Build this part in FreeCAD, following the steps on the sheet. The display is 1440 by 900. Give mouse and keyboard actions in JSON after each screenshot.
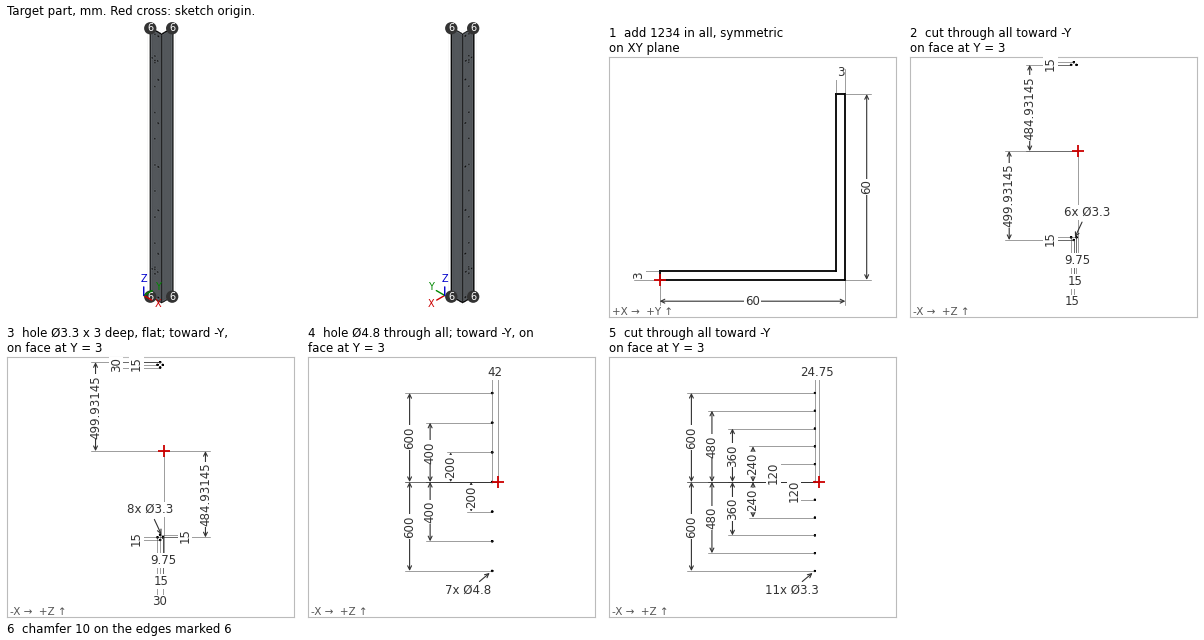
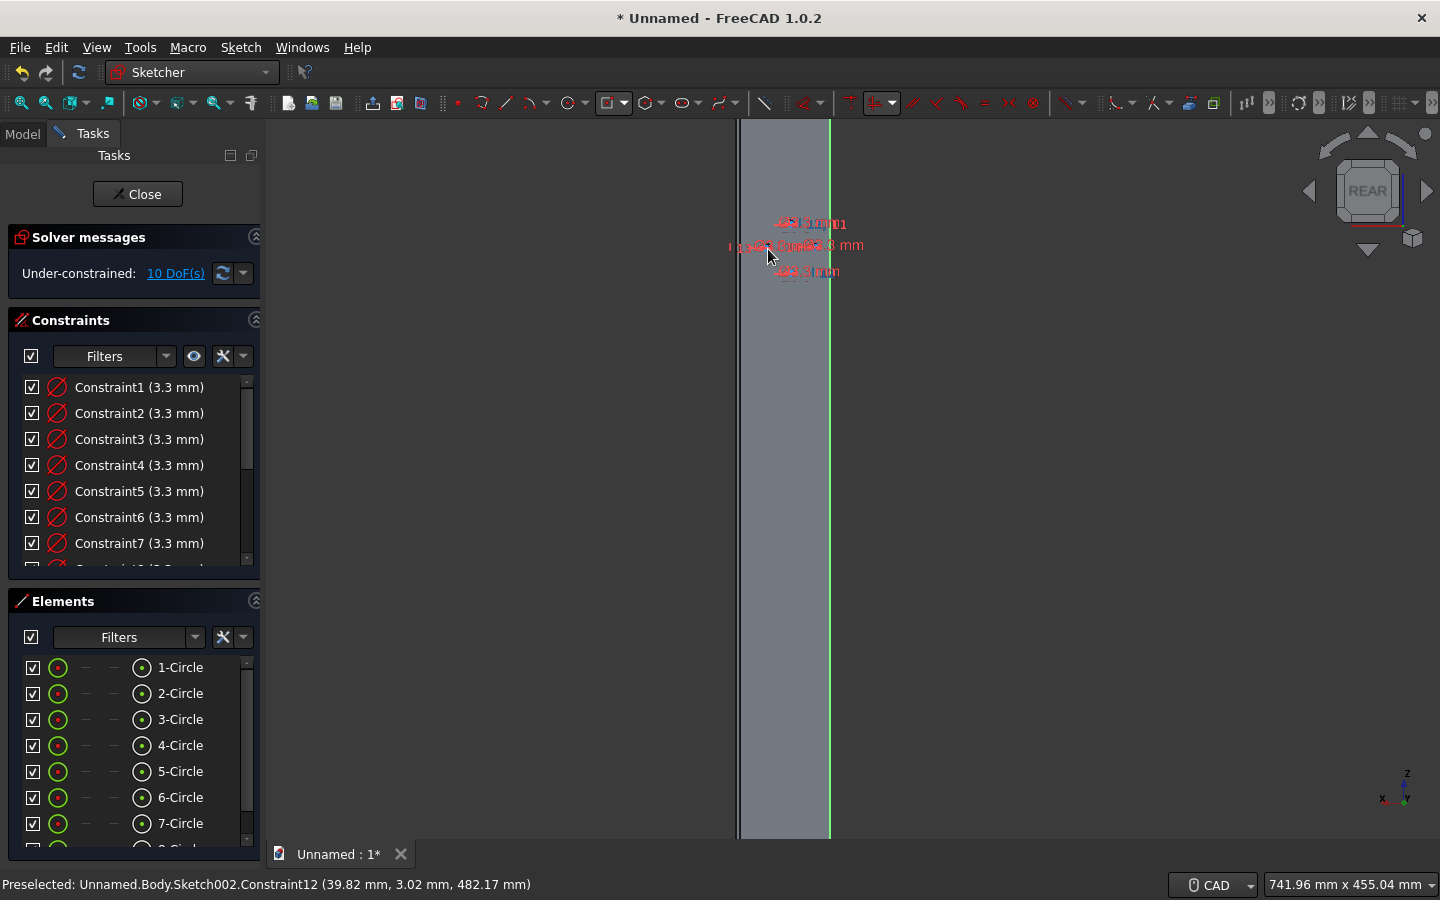
{"action": "left_click", "coordinate": [766, 248]}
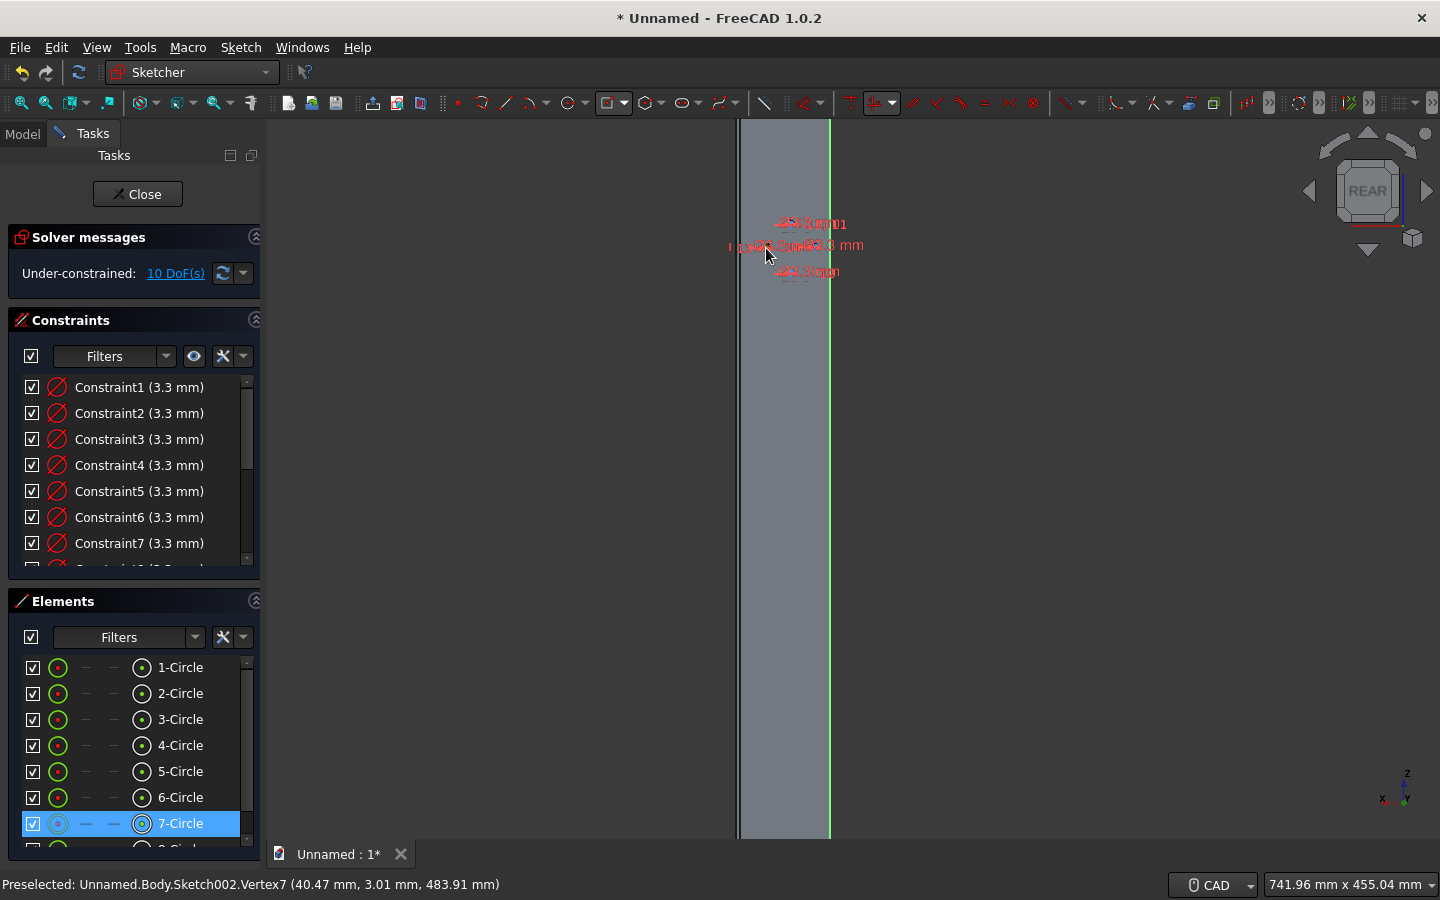
{"action": "left_click", "coordinate": [815, 247]}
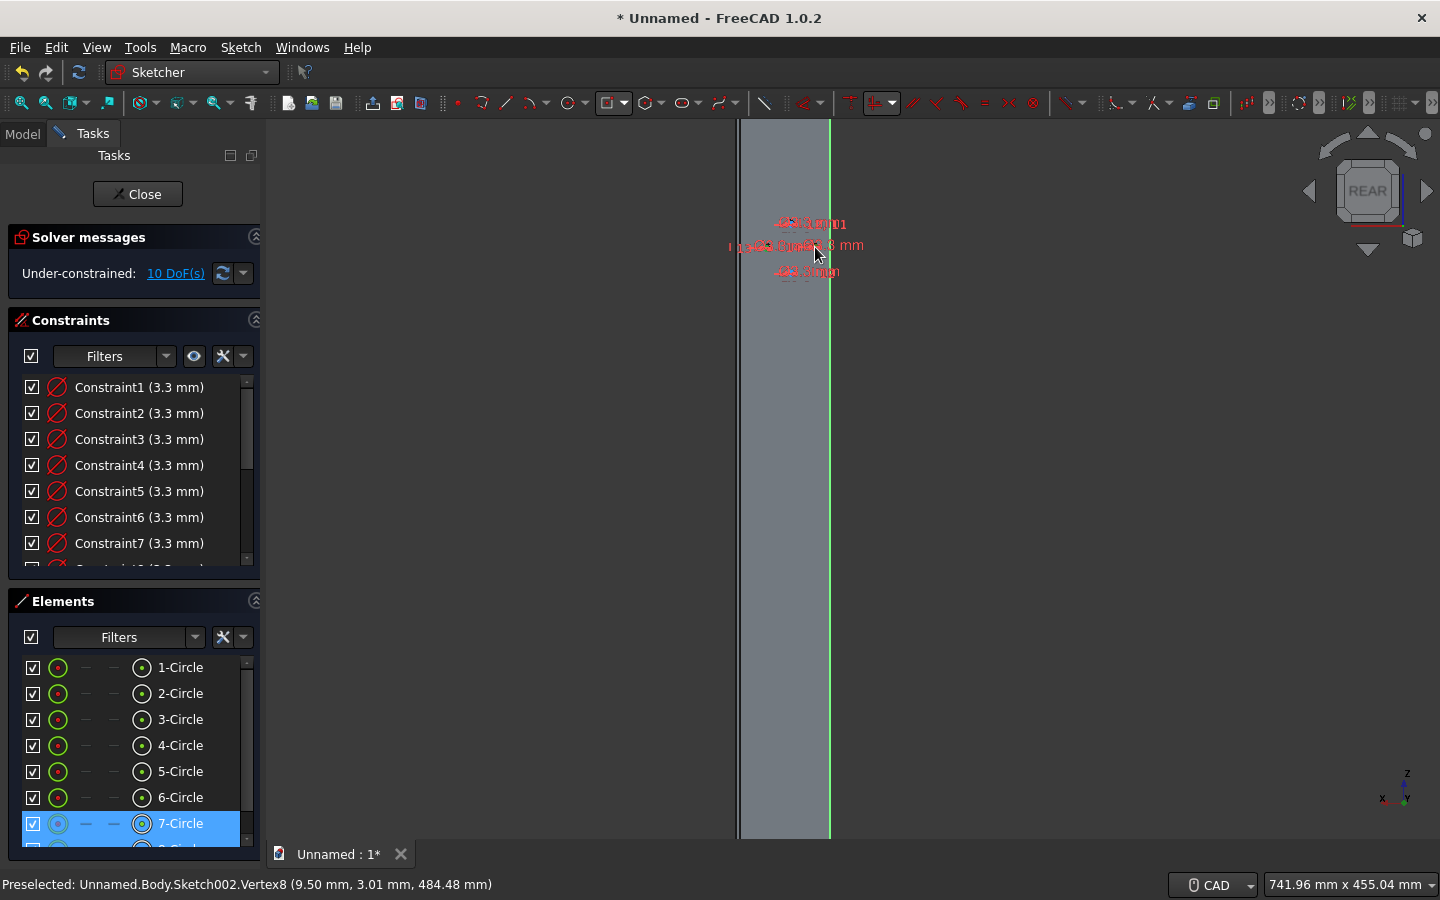
{"action": "left_click", "coordinate": [894, 104]}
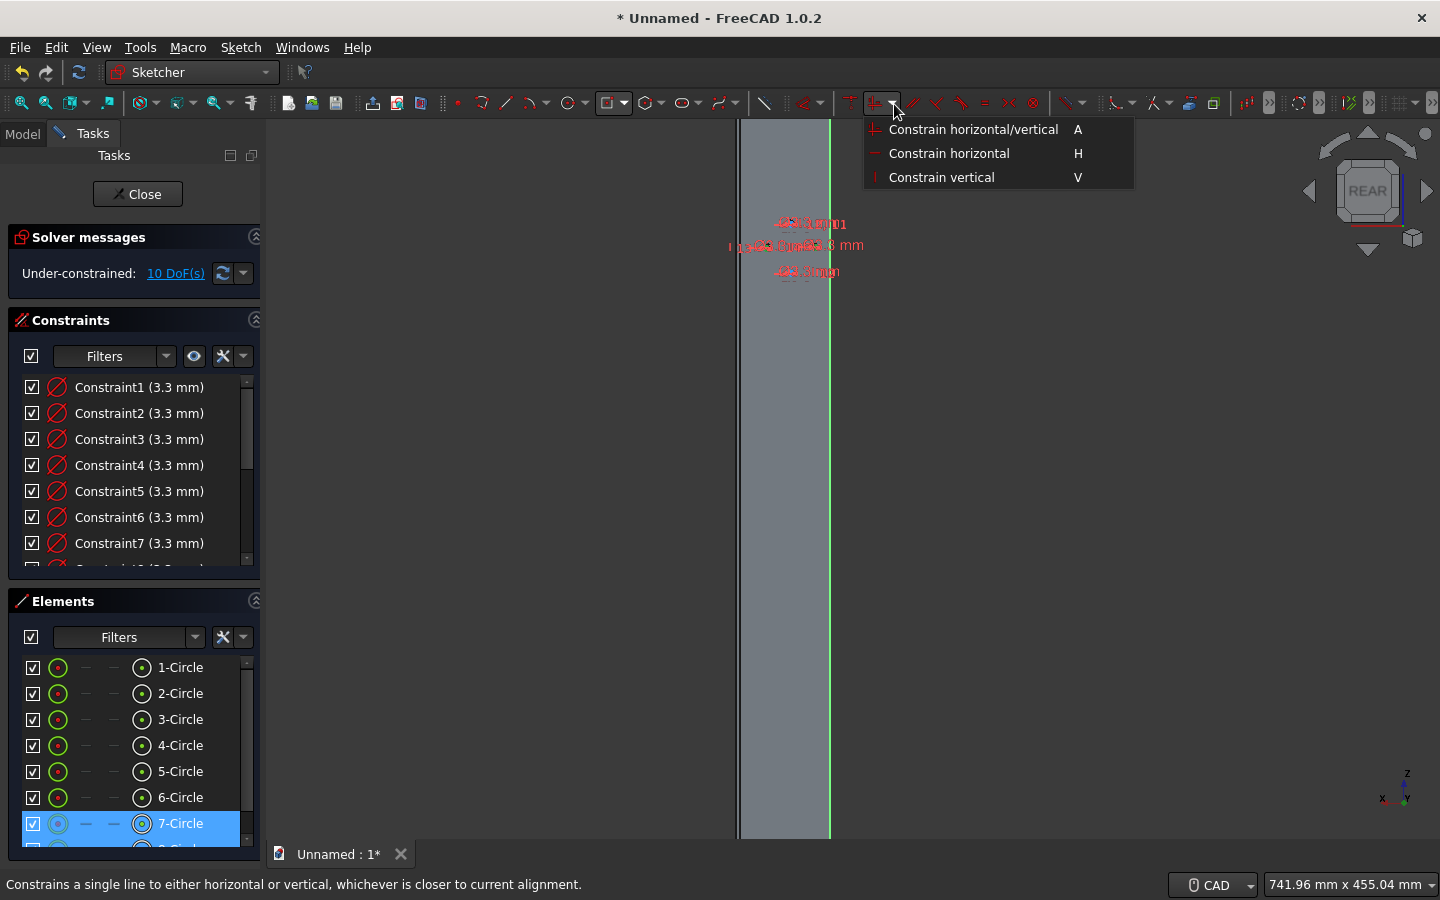
{"action": "left_click", "coordinate": [999, 153]}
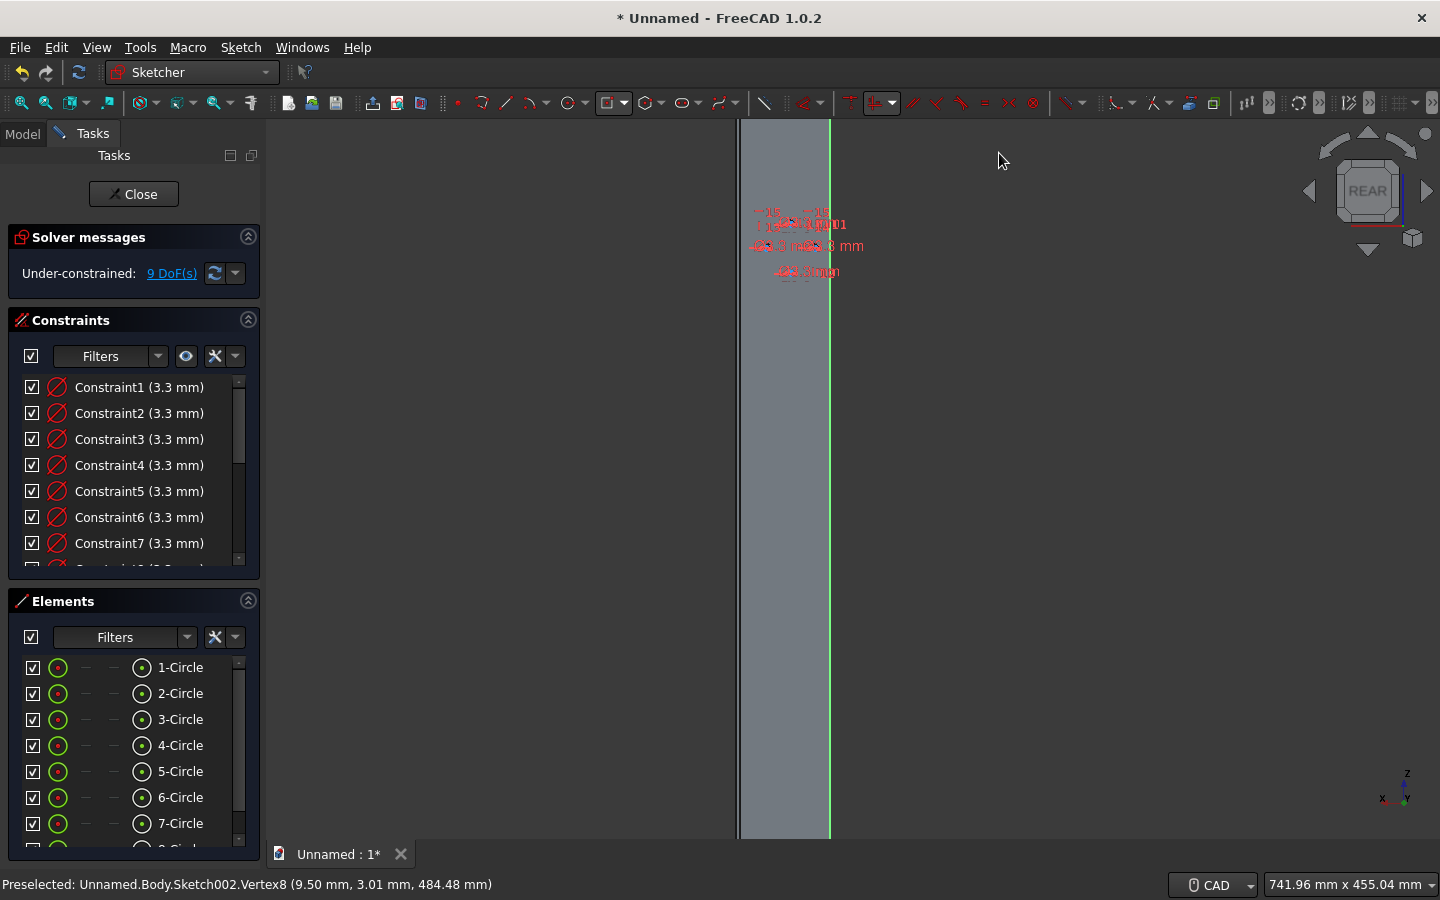
{"action": "left_click", "coordinate": [804, 104]}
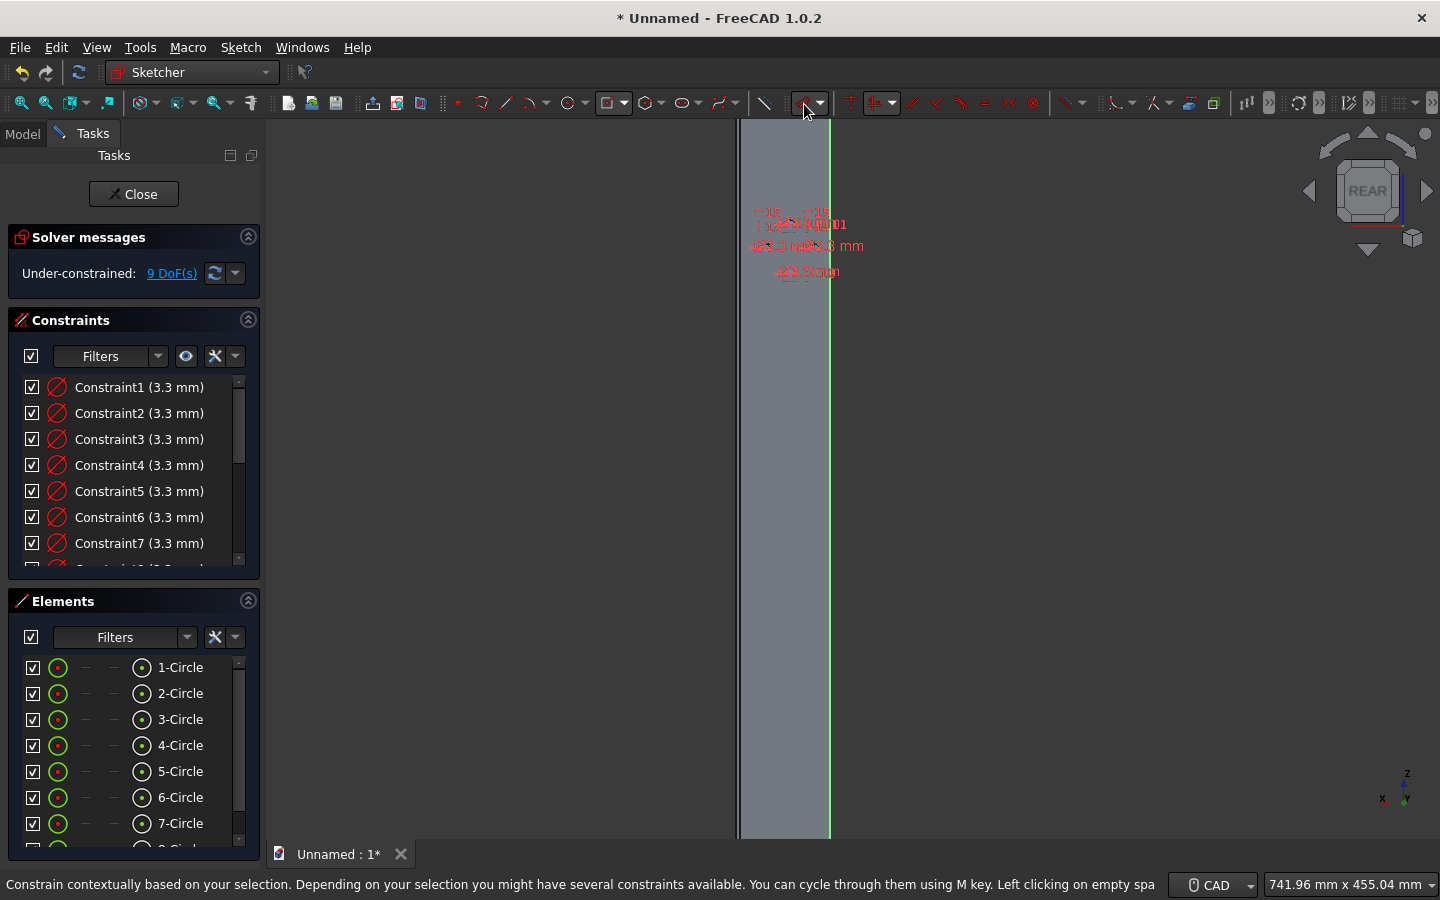
{"action": "scroll", "coordinate": [779, 248], "scroll_direction": "down", "scroll_amount": 6}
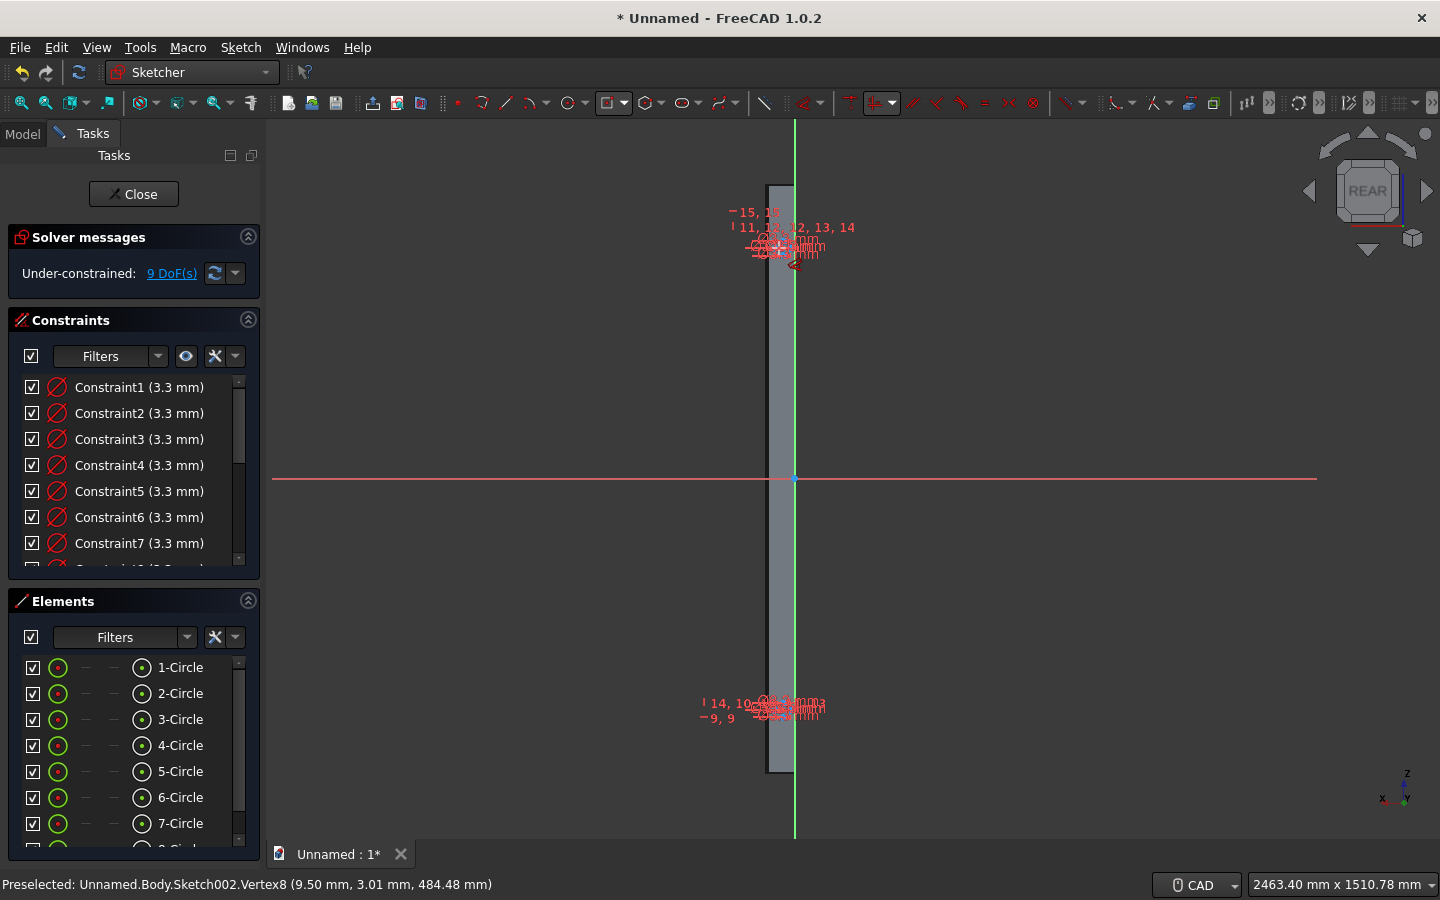
{"action": "scroll", "coordinate": [790, 710], "scroll_direction": "up", "scroll_amount": 6}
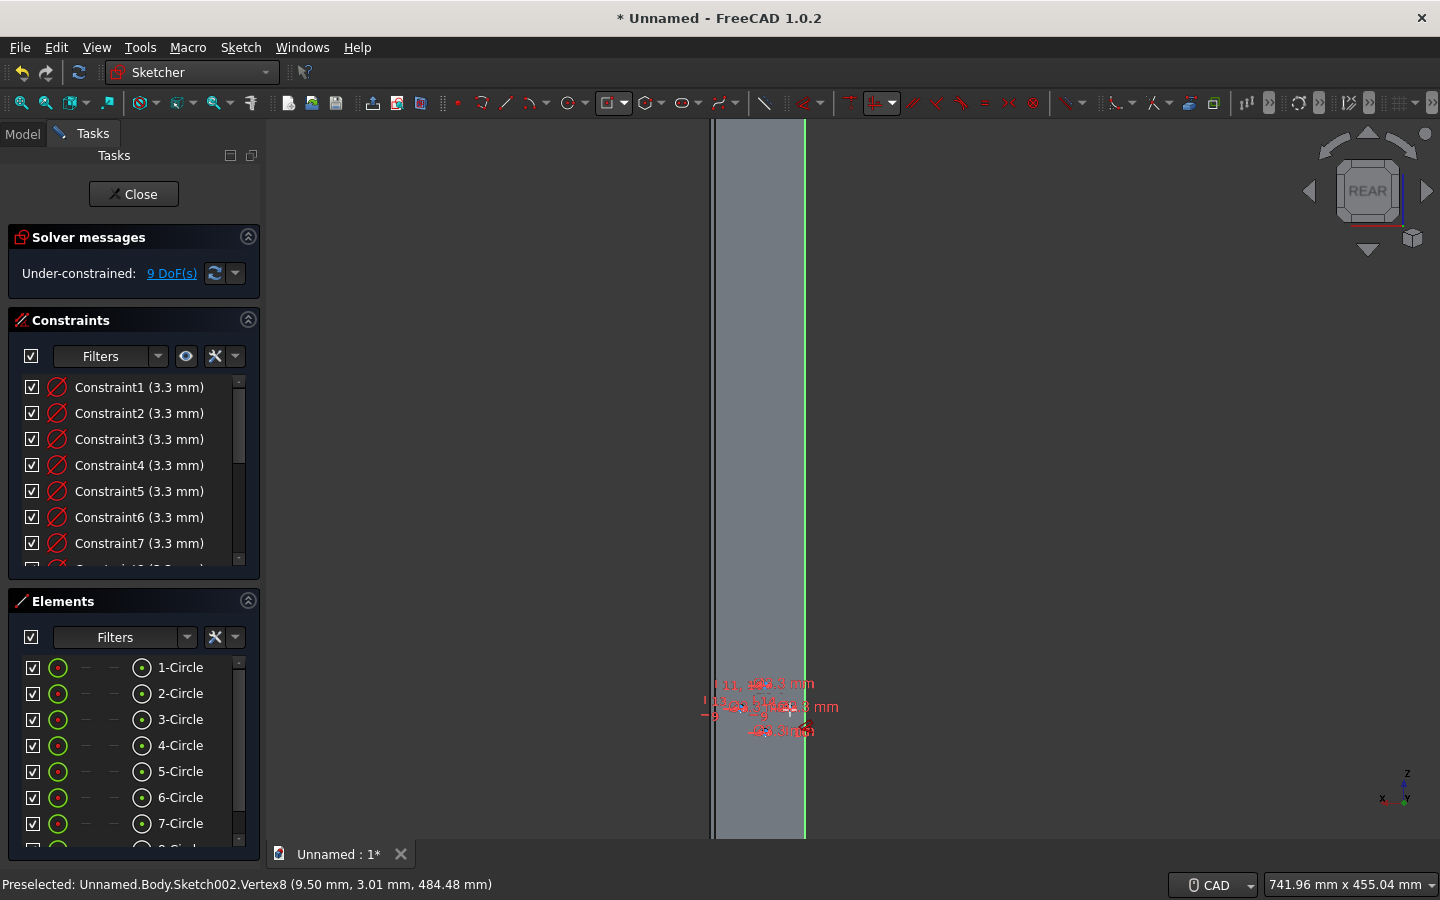
{"action": "left_click", "coordinate": [790, 709]}